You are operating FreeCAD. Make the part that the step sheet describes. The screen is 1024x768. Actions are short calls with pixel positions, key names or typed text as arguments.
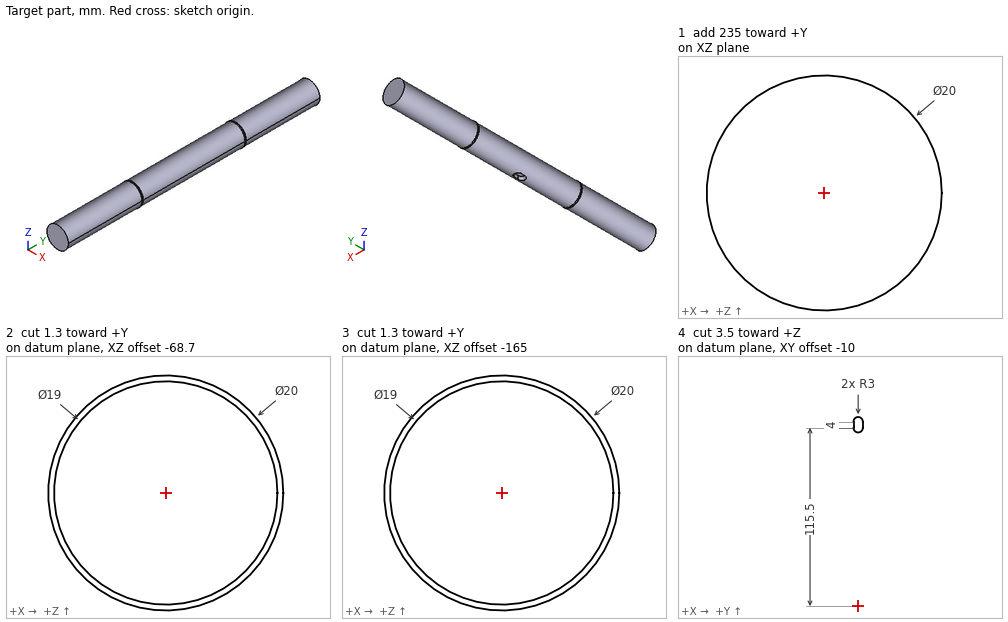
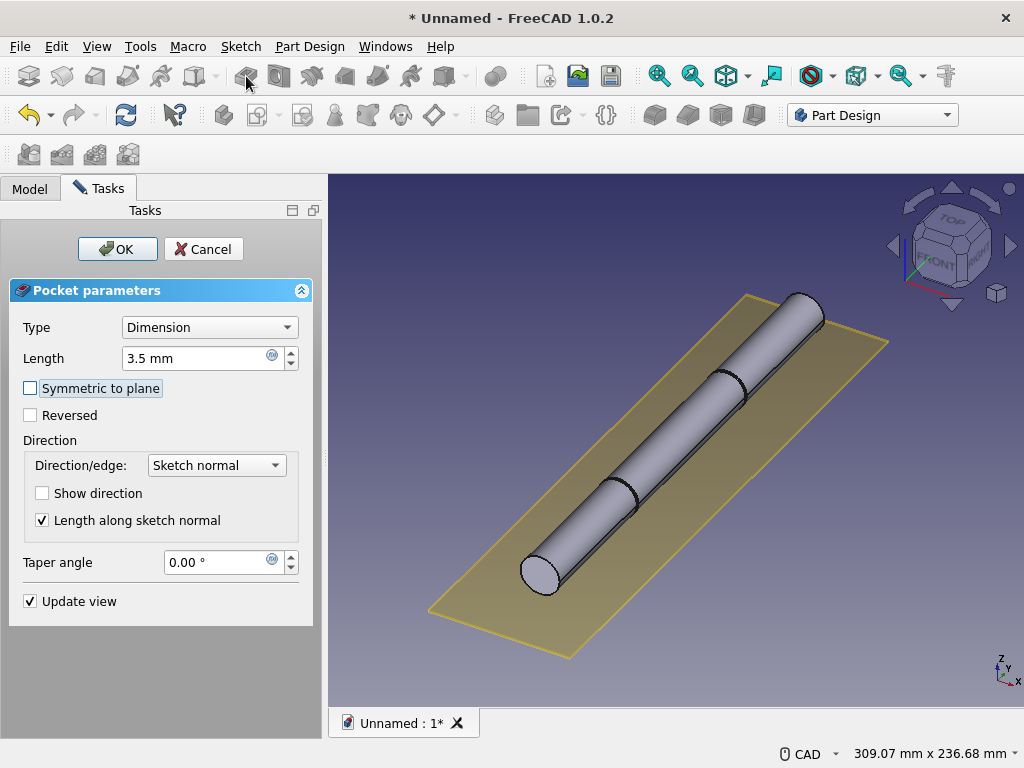
click(31, 415)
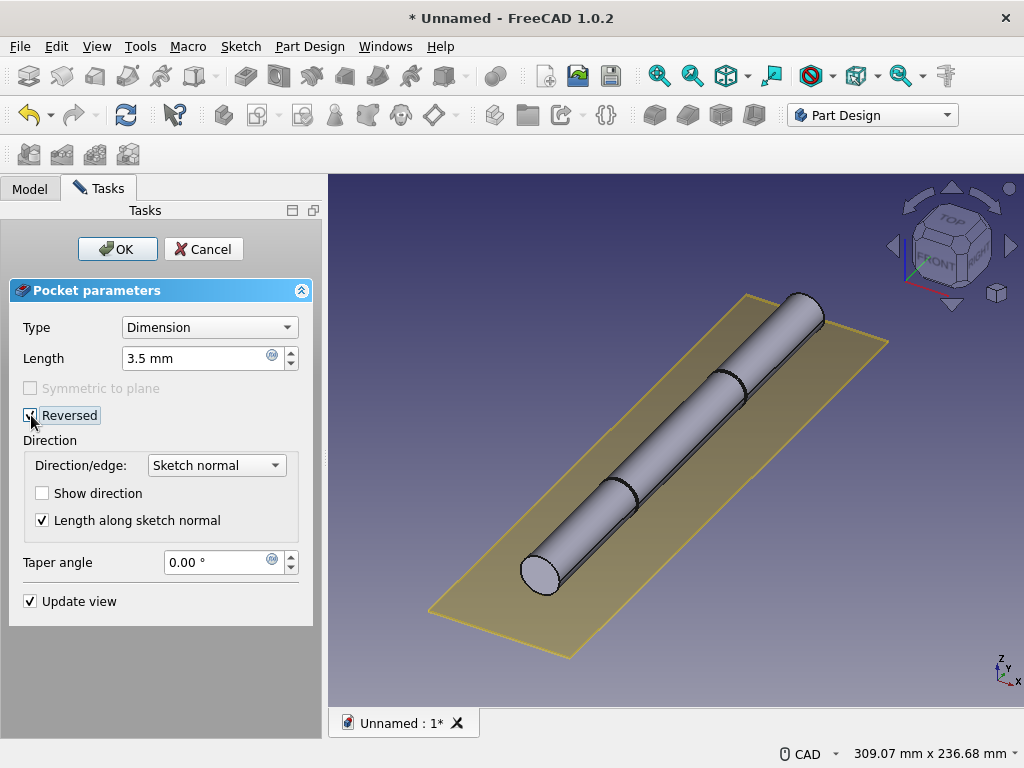
click(118, 249)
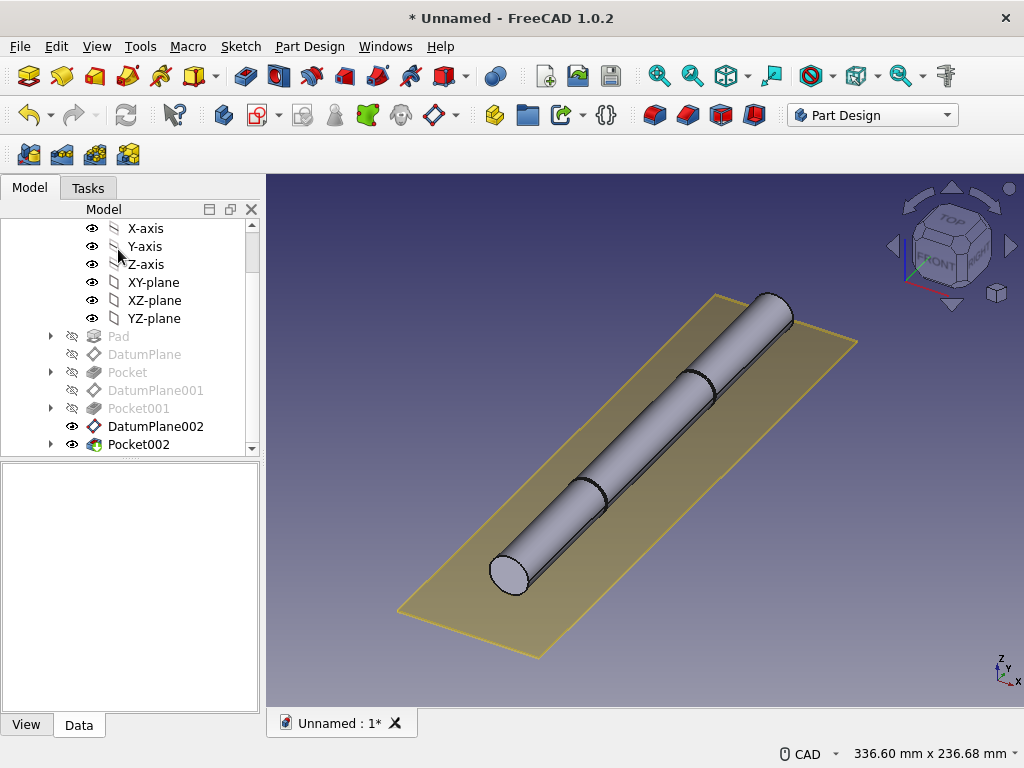
click(117, 426)
key(space)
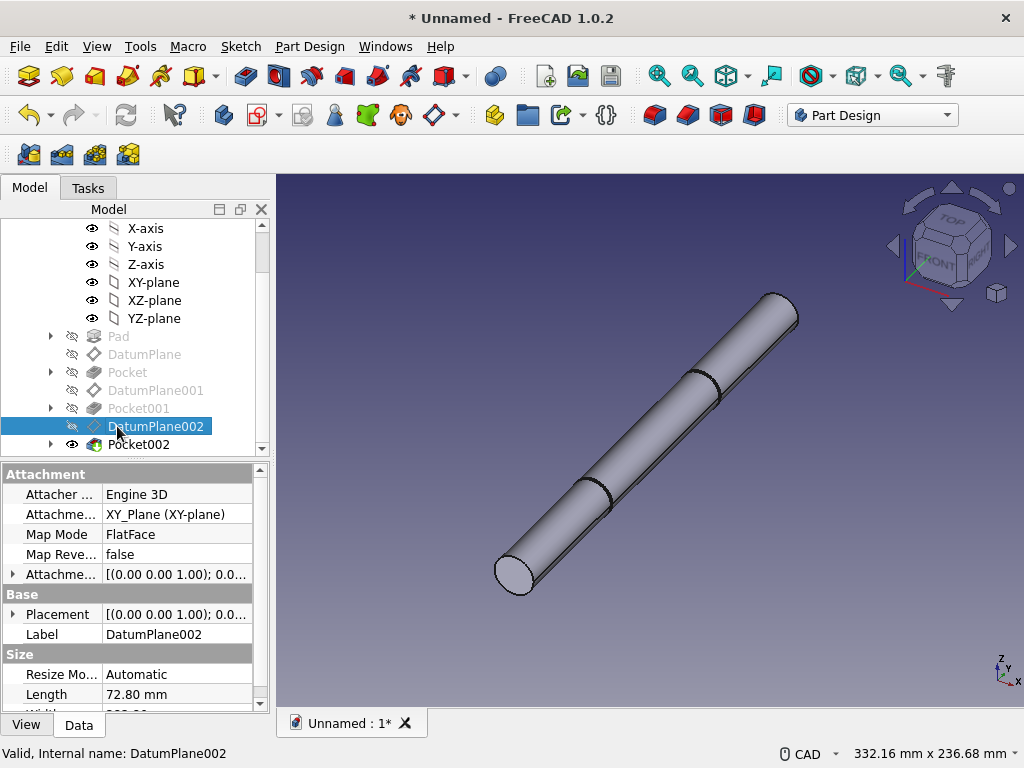
key(0)